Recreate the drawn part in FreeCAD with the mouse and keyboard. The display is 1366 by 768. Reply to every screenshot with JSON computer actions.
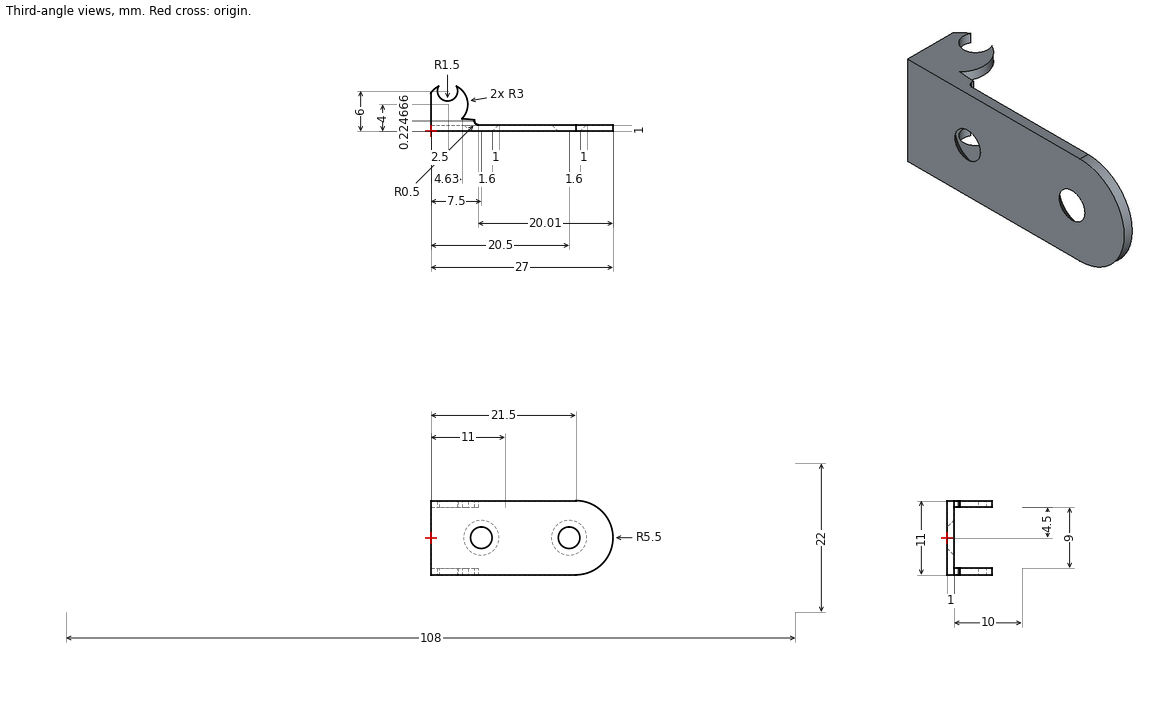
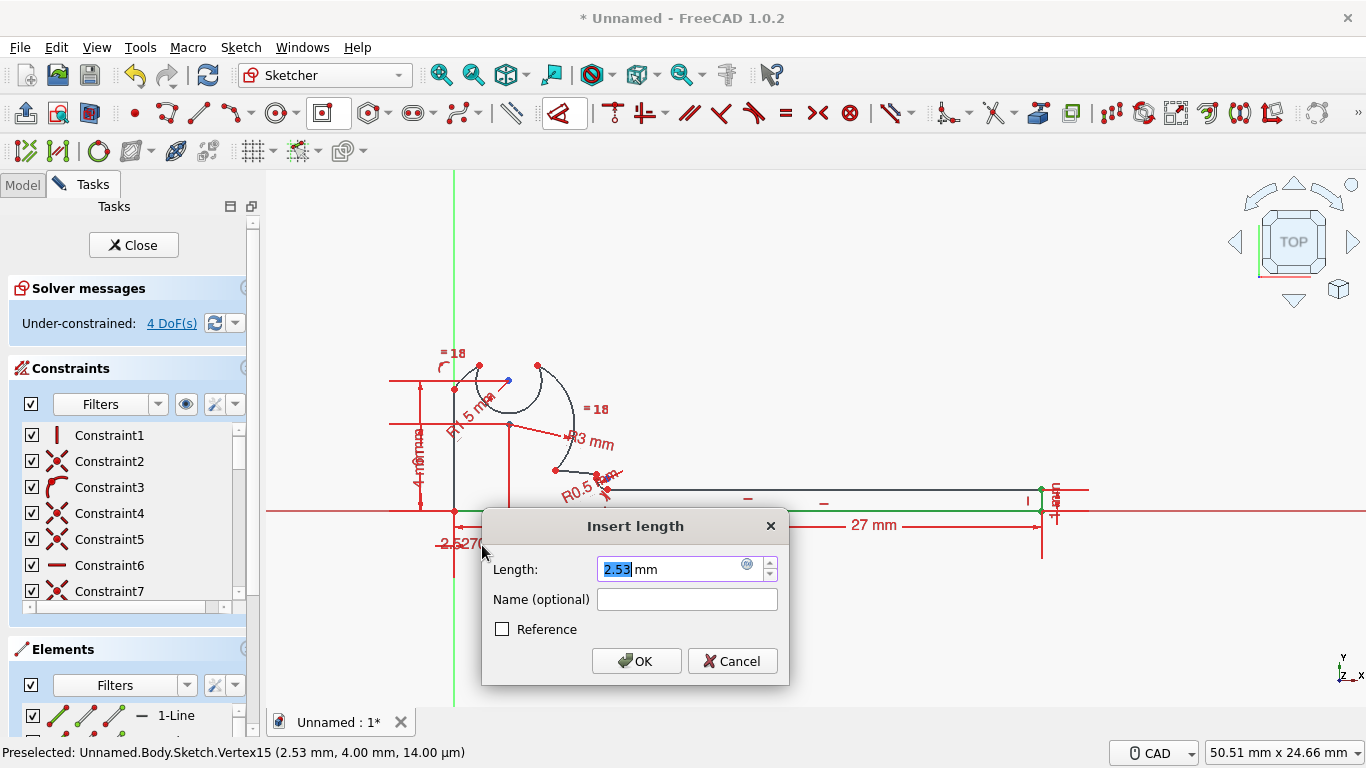
{"action": "type", "text": "2.5"}
{"action": "key", "text": "Return"}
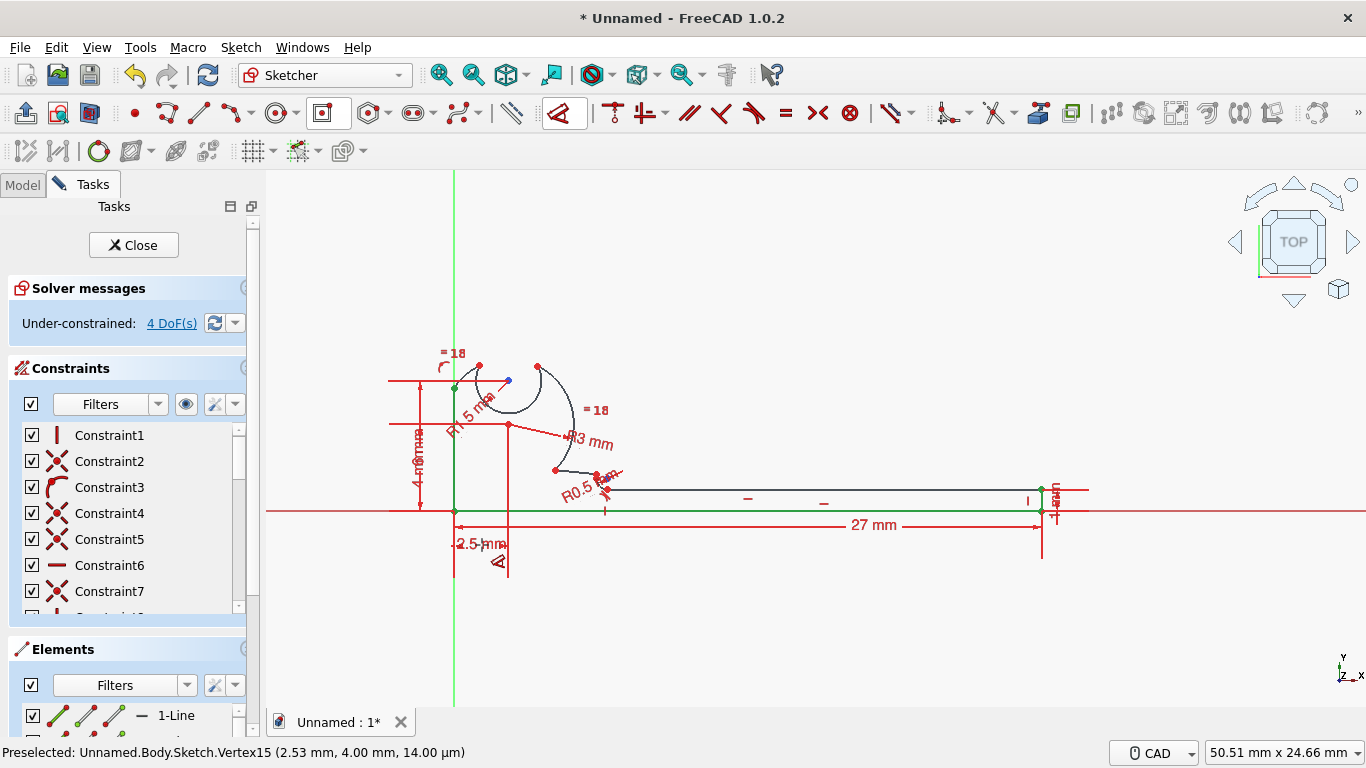
{"action": "left_click", "coordinate": [509, 381]}
{"action": "left_click", "coordinate": [481, 347]}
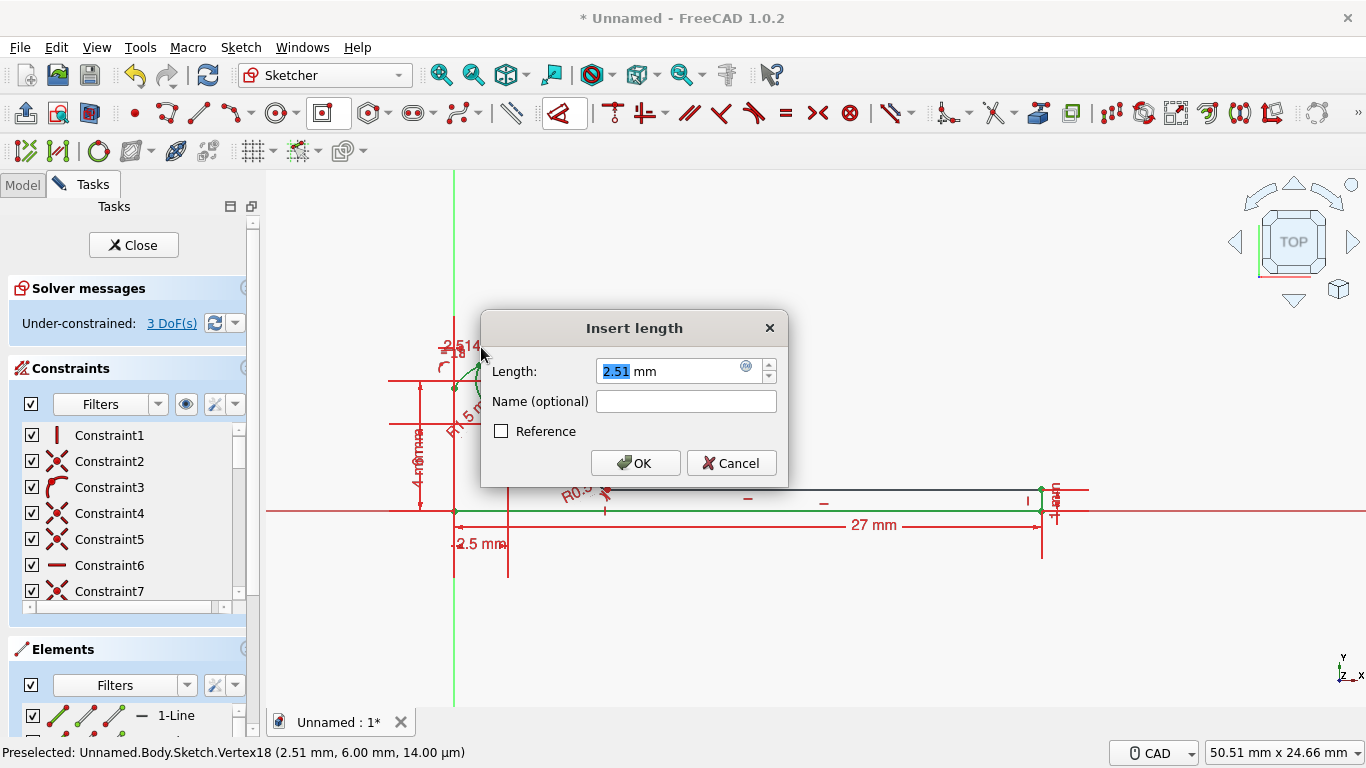
{"action": "type", "text": "2.5"}
{"action": "key", "text": "Return"}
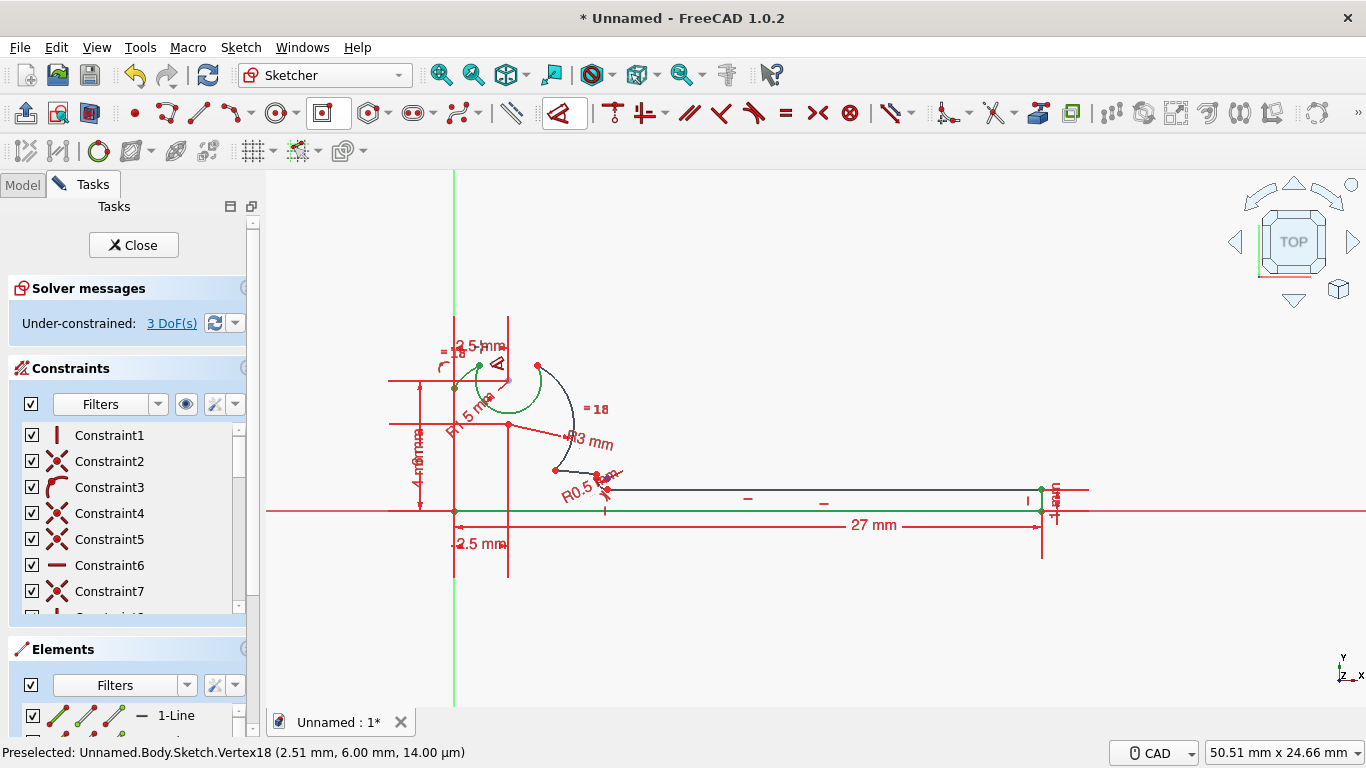
{"action": "left_click", "coordinate": [912, 490]}
{"action": "left_click", "coordinate": [825, 456]}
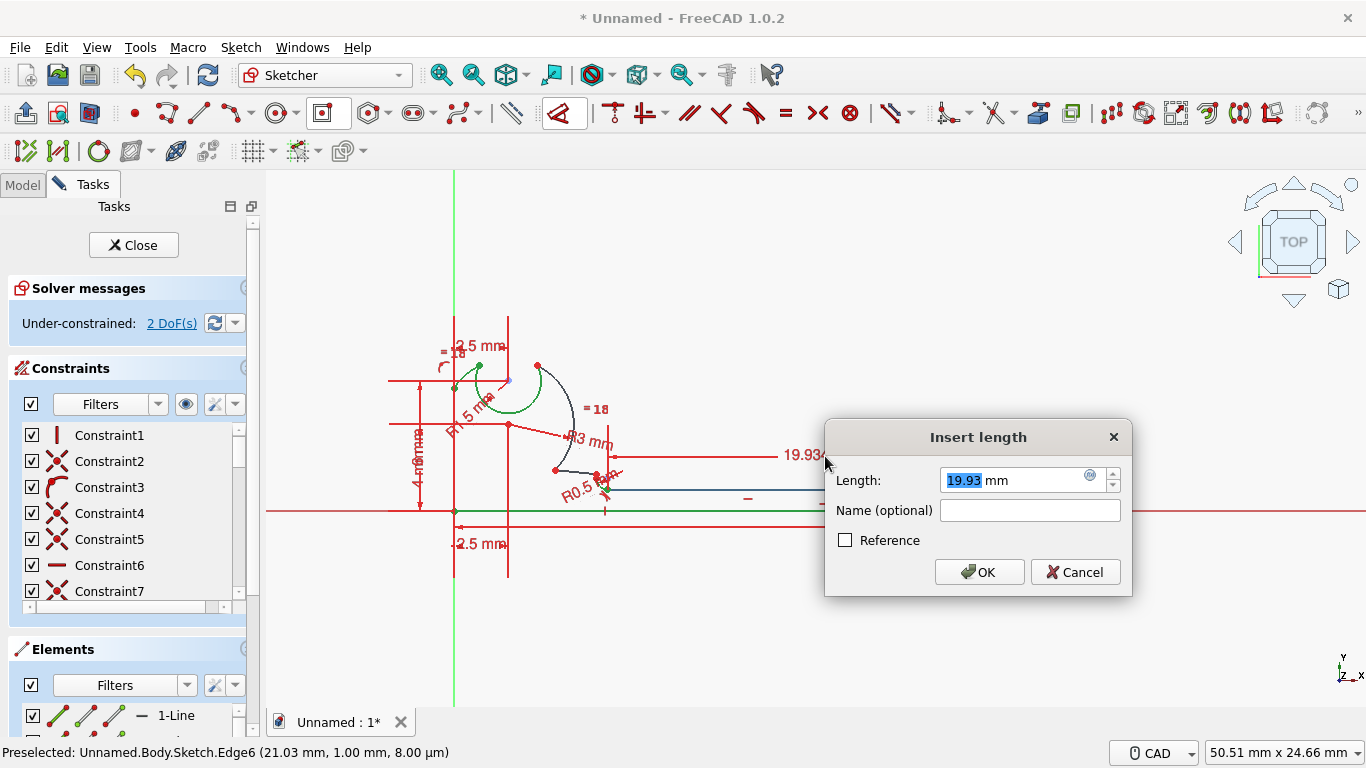
{"action": "type", "text": "20.01"}
{"action": "key", "text": "Return"}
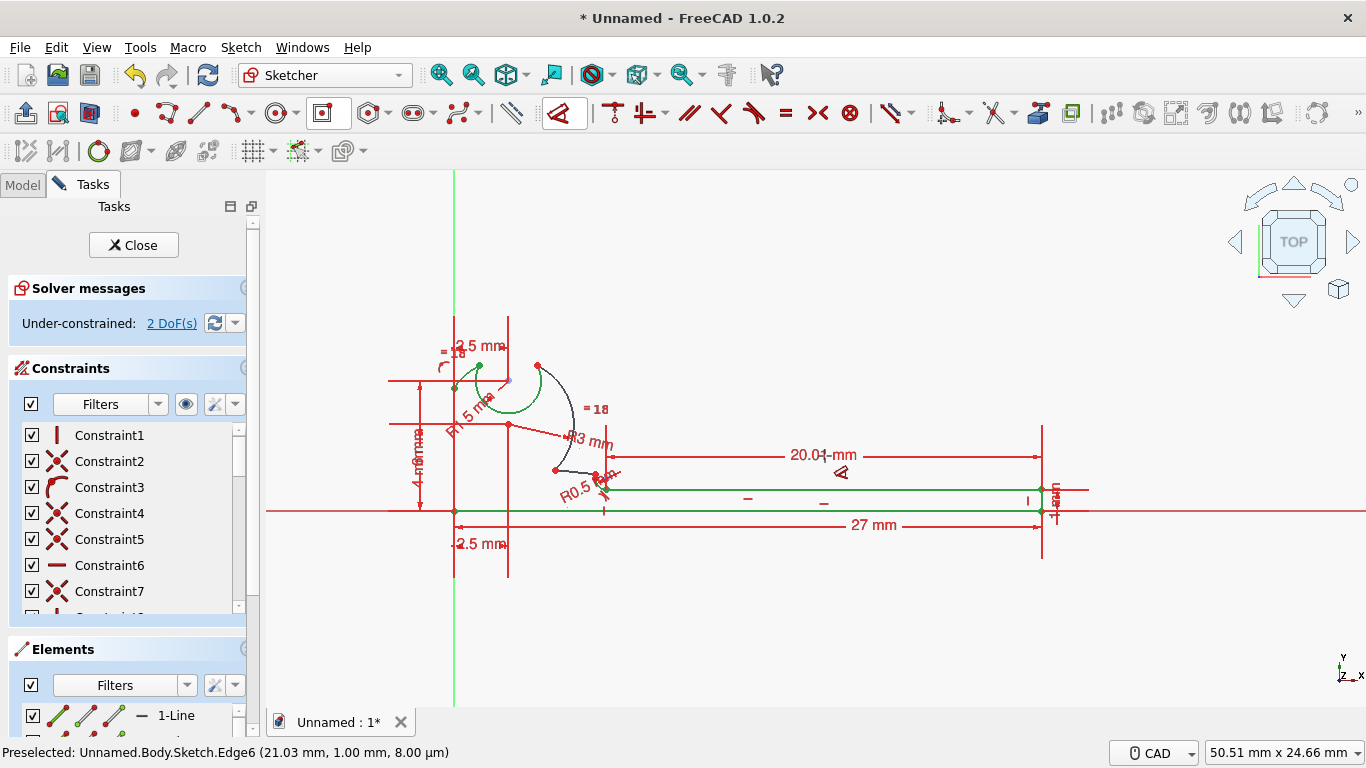
{"action": "left_click", "coordinate": [555, 470]}
{"action": "left_click", "coordinate": [505, 436]}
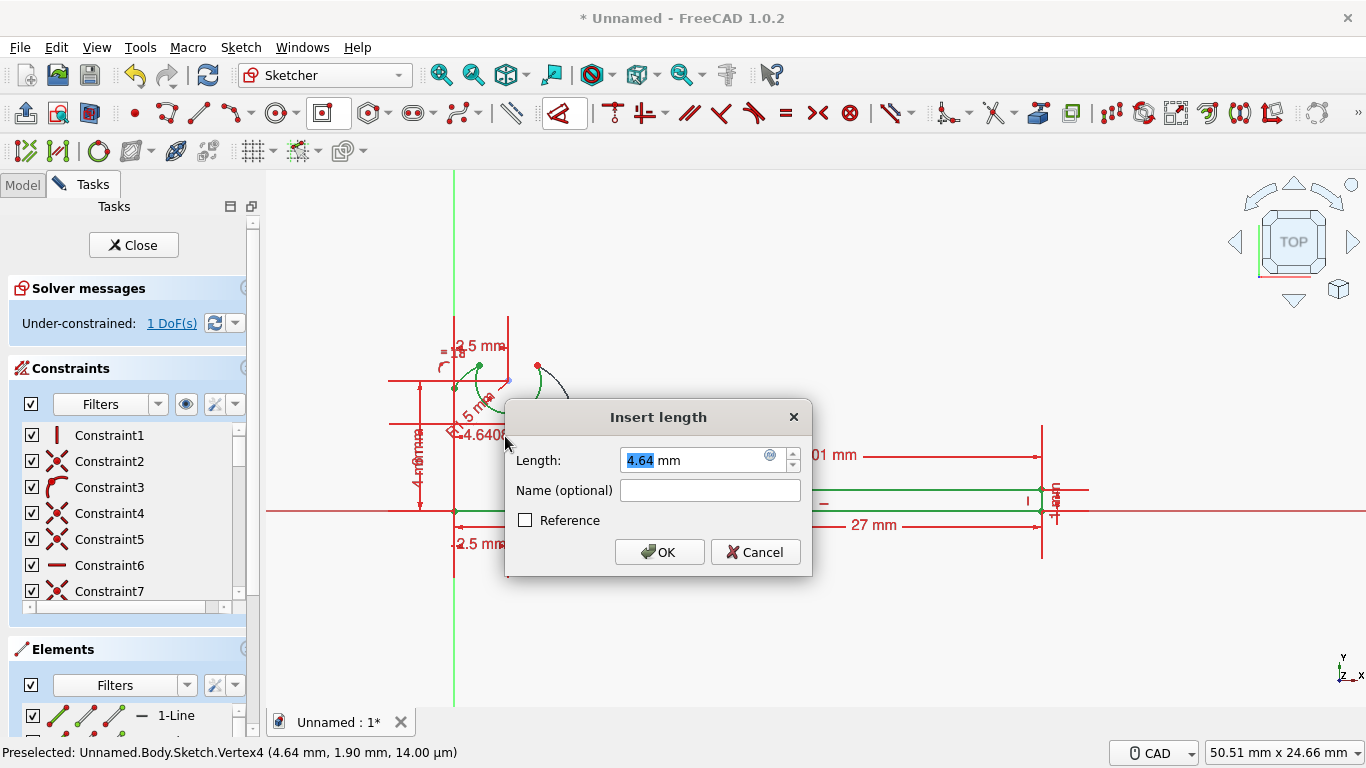
{"action": "type", "text": "4.63"}
{"action": "key", "text": "Return"}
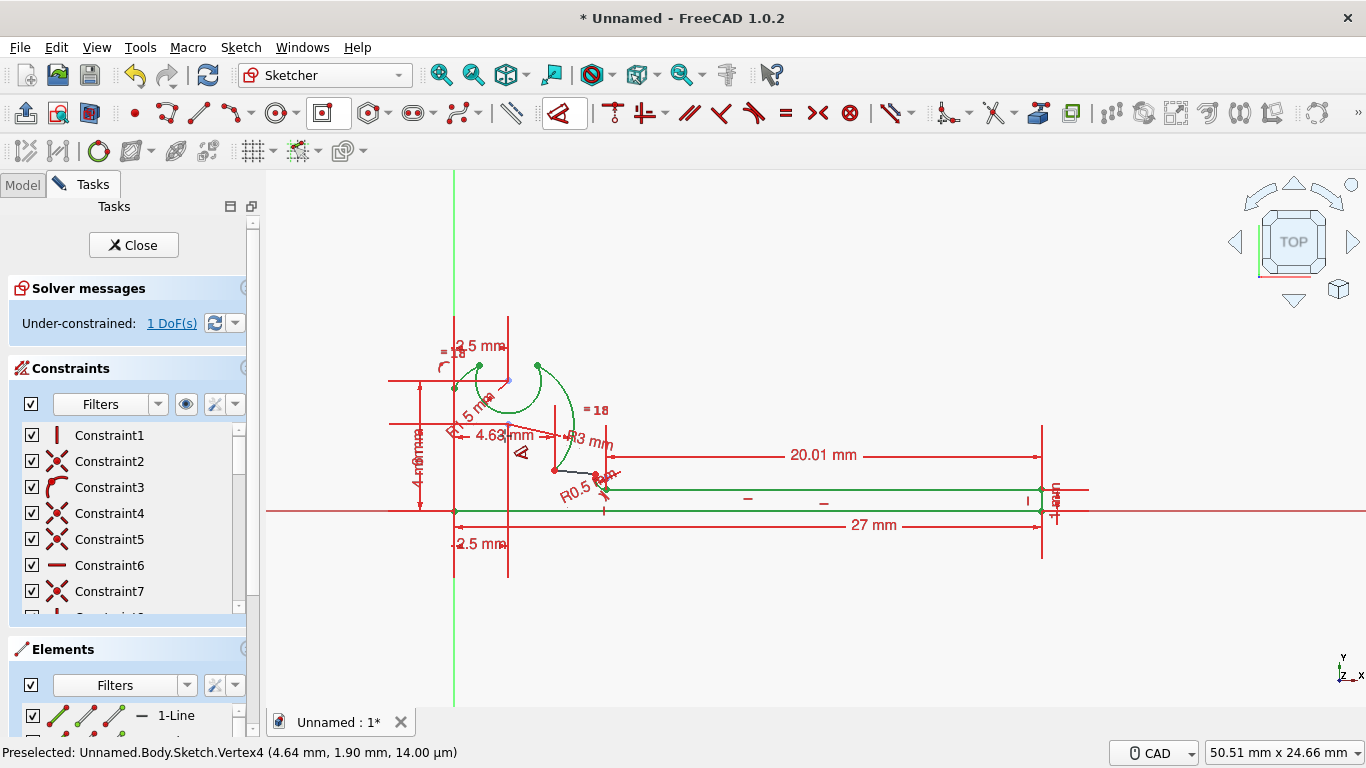
{"action": "scroll", "coordinate": [595, 477], "scroll_direction": "up", "scroll_amount": 11}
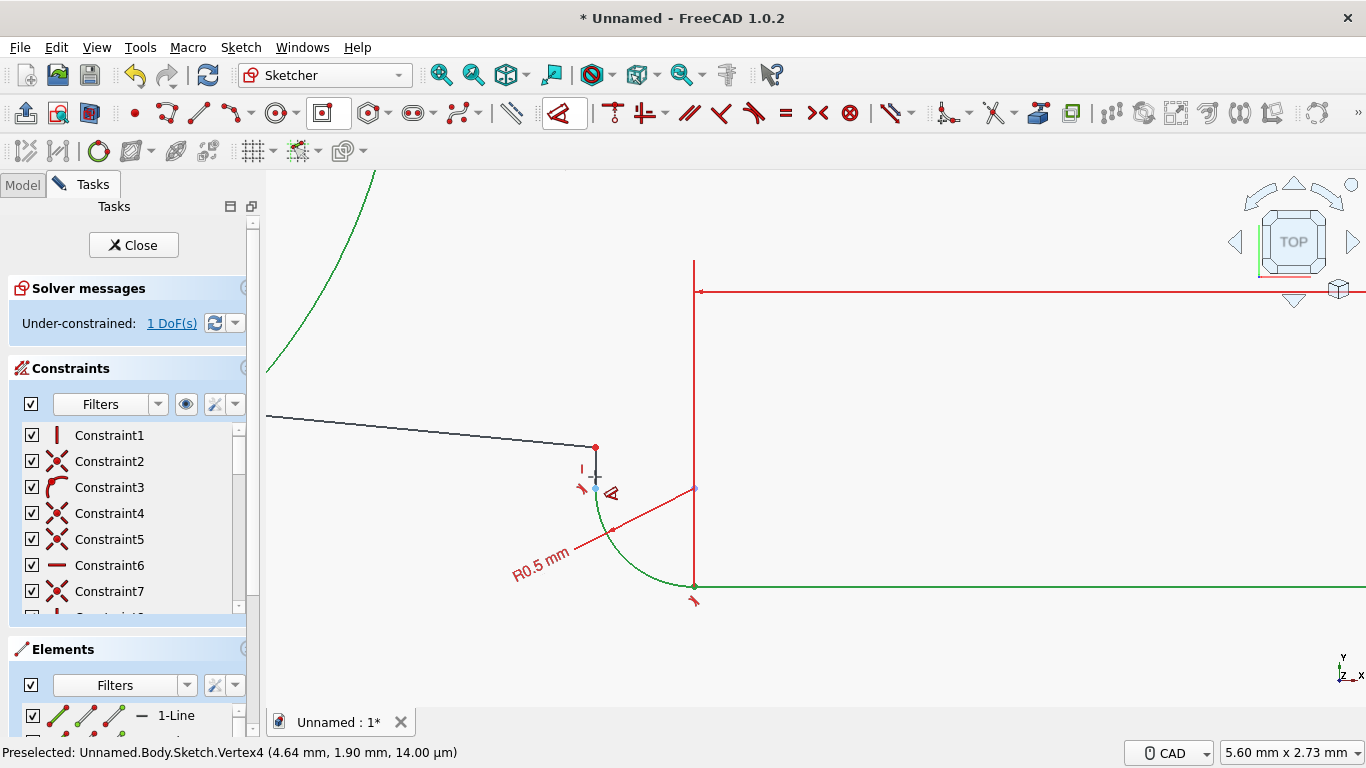
{"action": "left_click", "coordinate": [596, 468]}
{"action": "left_click", "coordinate": [562, 468]}